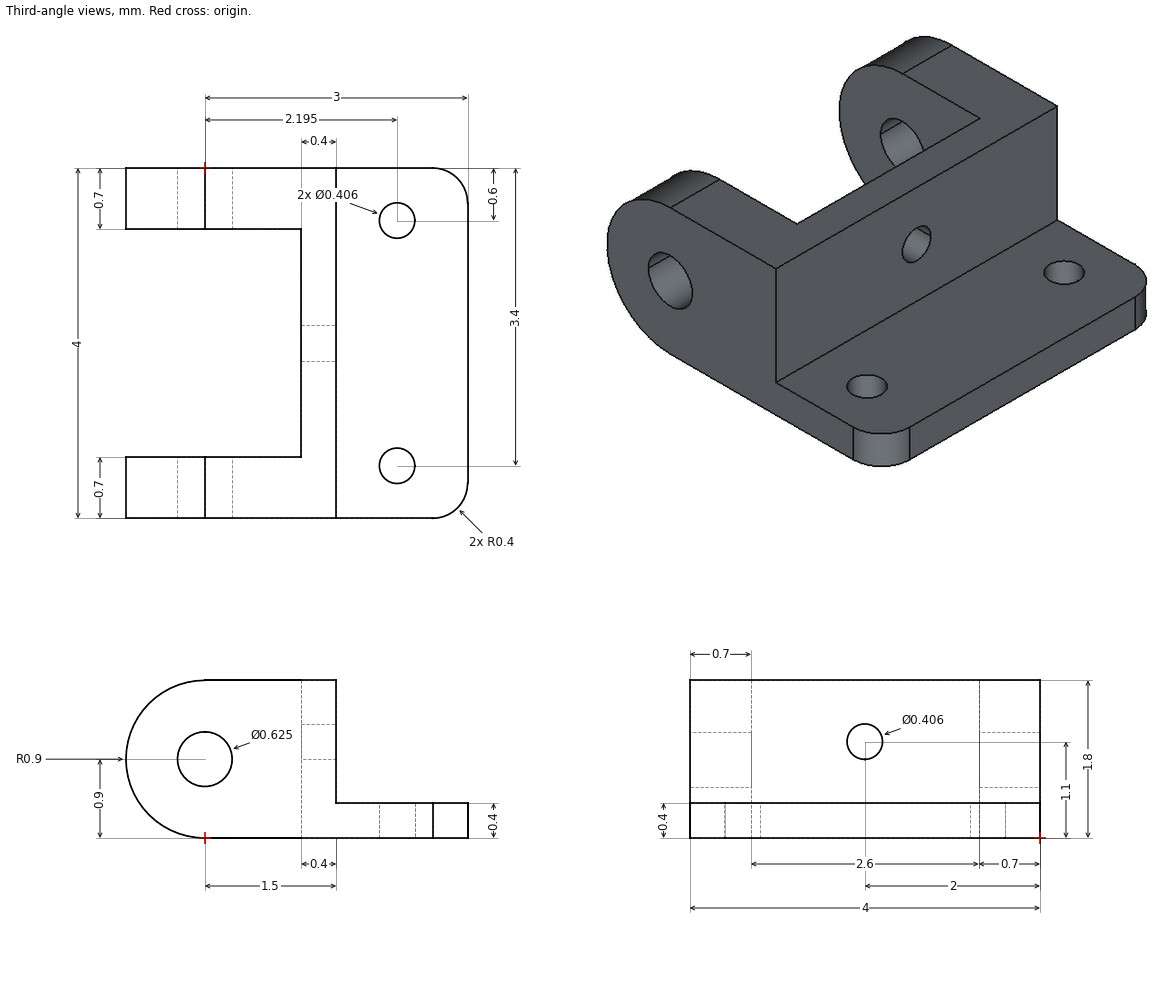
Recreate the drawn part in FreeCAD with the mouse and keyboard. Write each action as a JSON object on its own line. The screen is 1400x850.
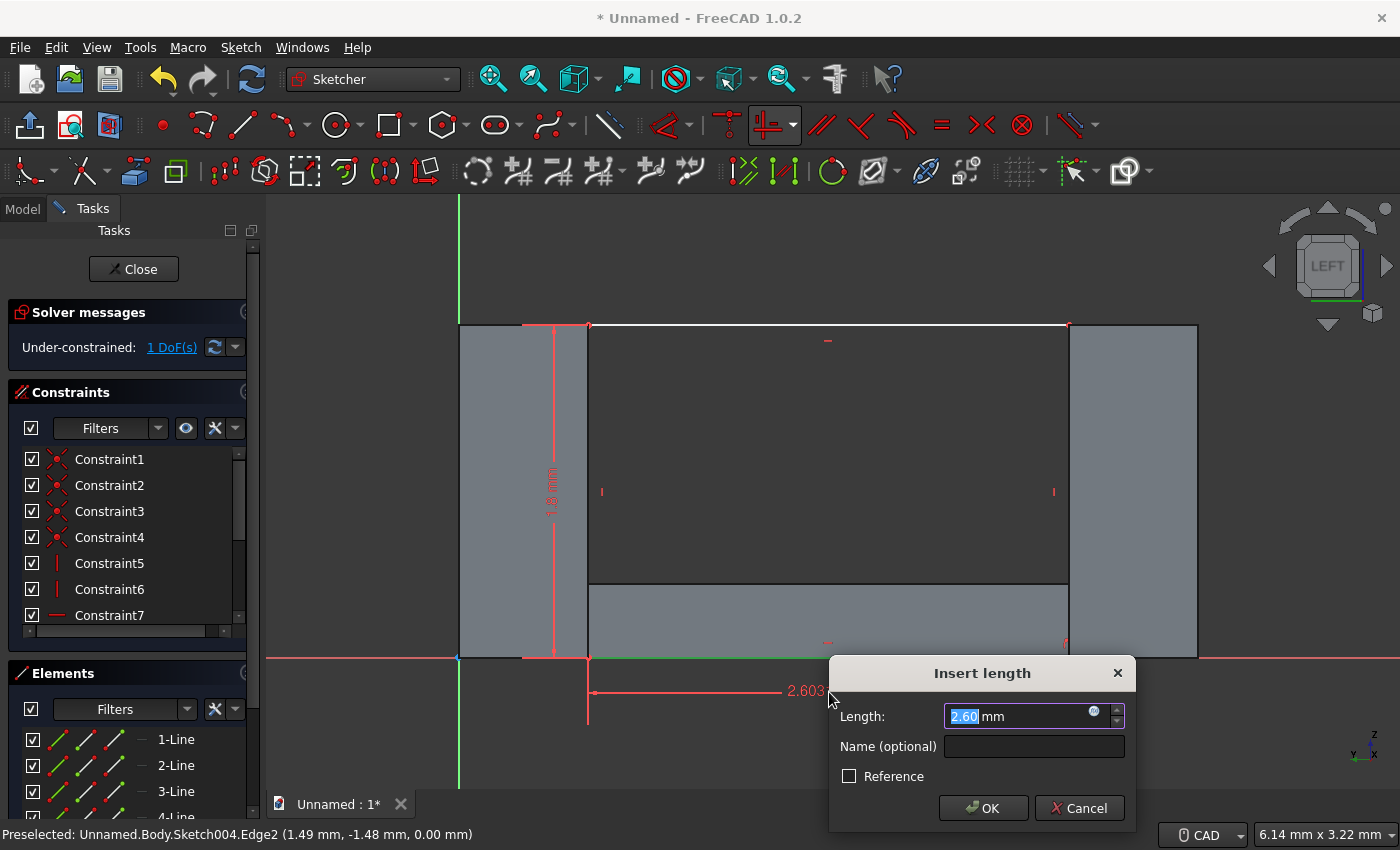
{"action": "type", "text": "2.6"}
{"action": "key", "text": "Return"}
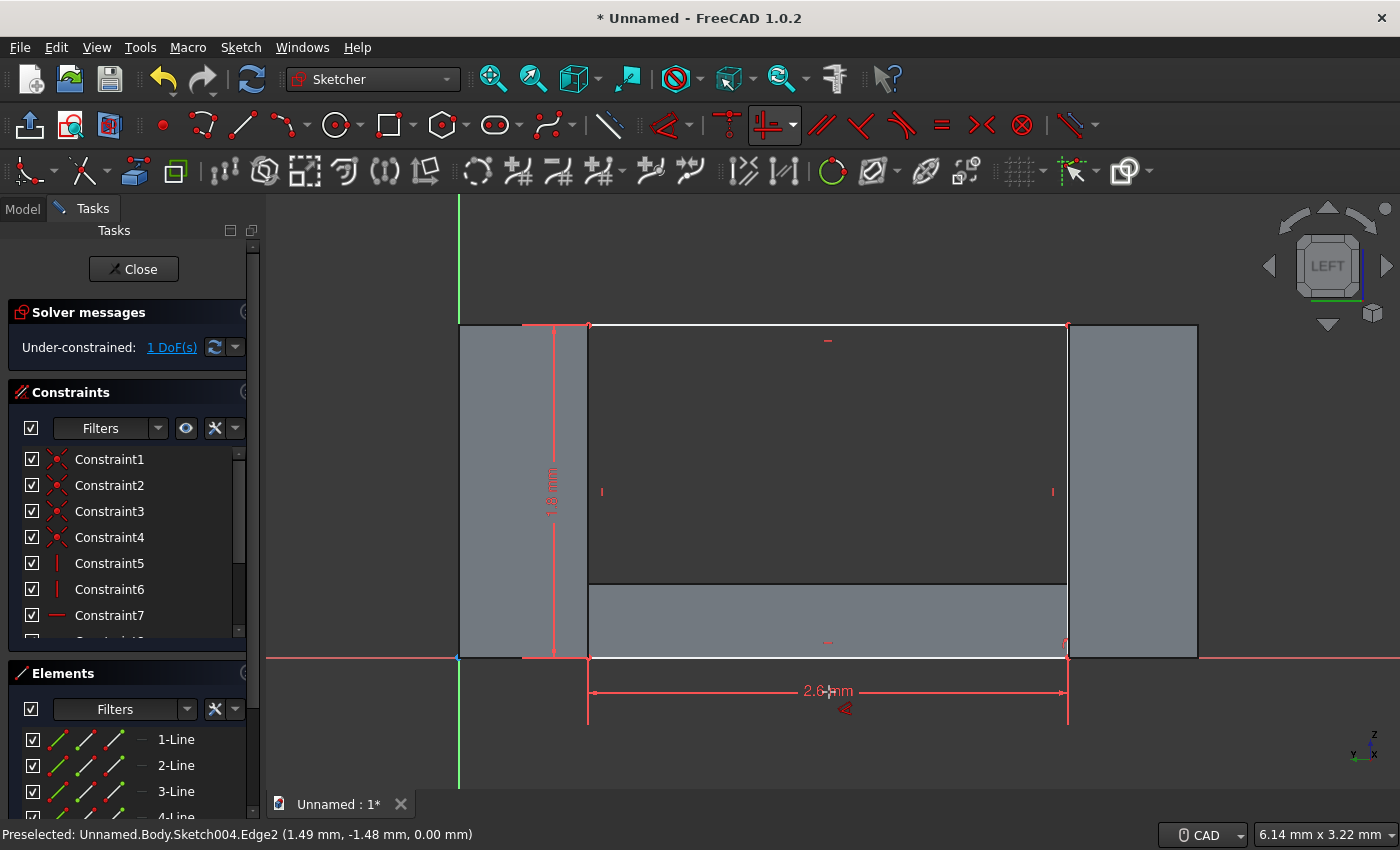
{"action": "left_click", "coordinate": [588, 325]}
{"action": "left_click", "coordinate": [523, 692]}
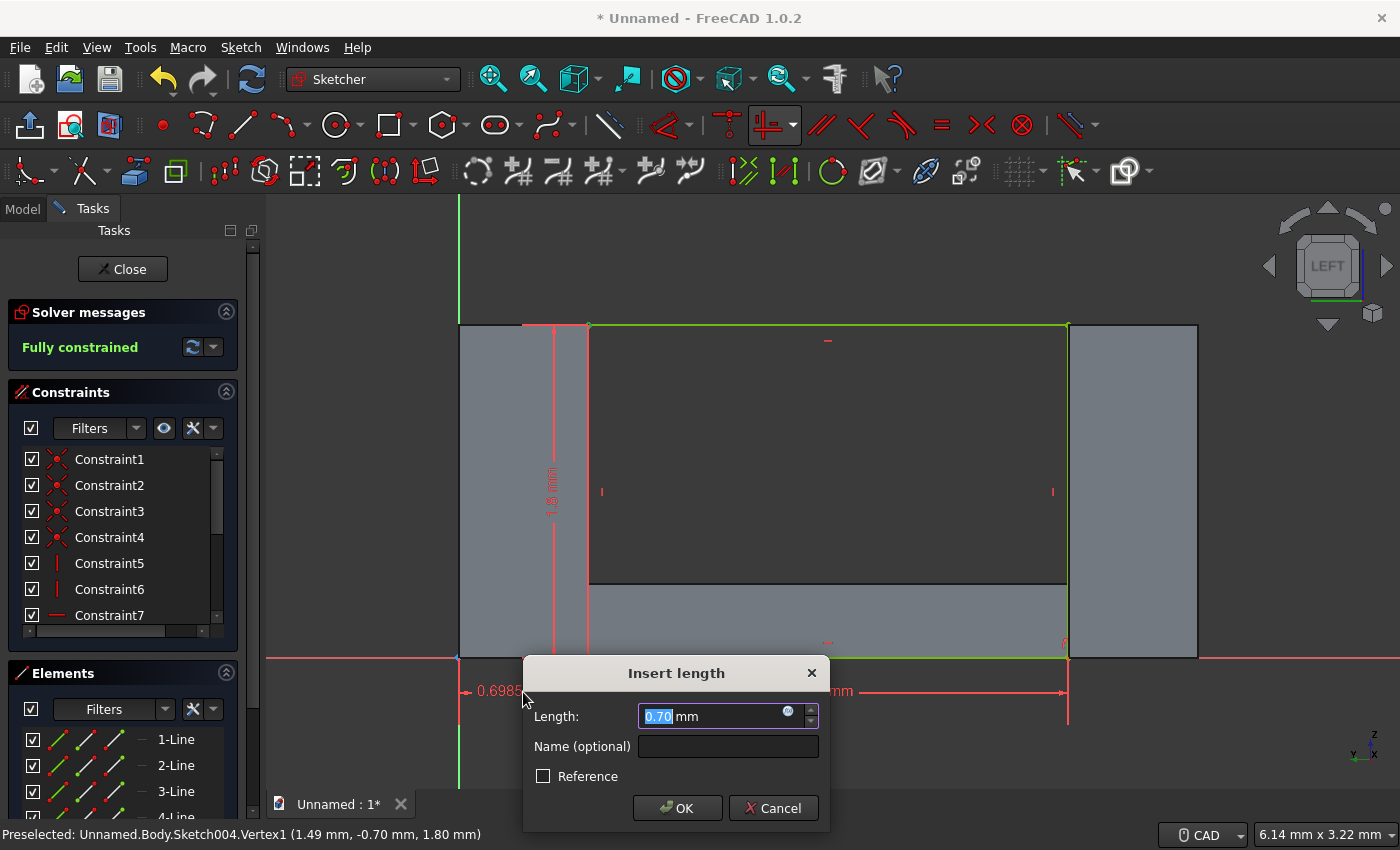
{"action": "type", "text": "0.7"}
{"action": "key", "text": "Return"}
{"action": "key", "text": "Escape"}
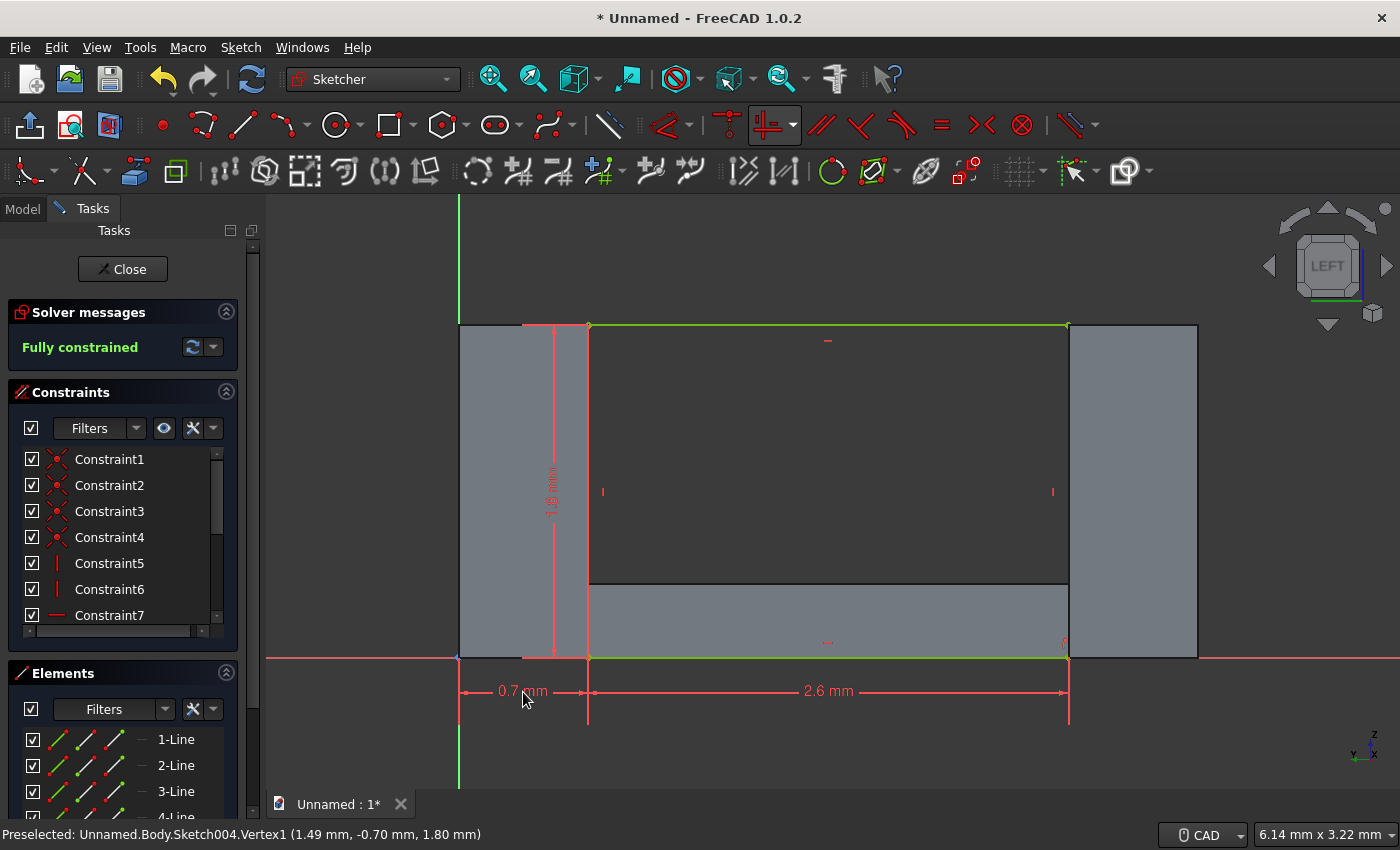
{"action": "left_click", "coordinate": [123, 269]}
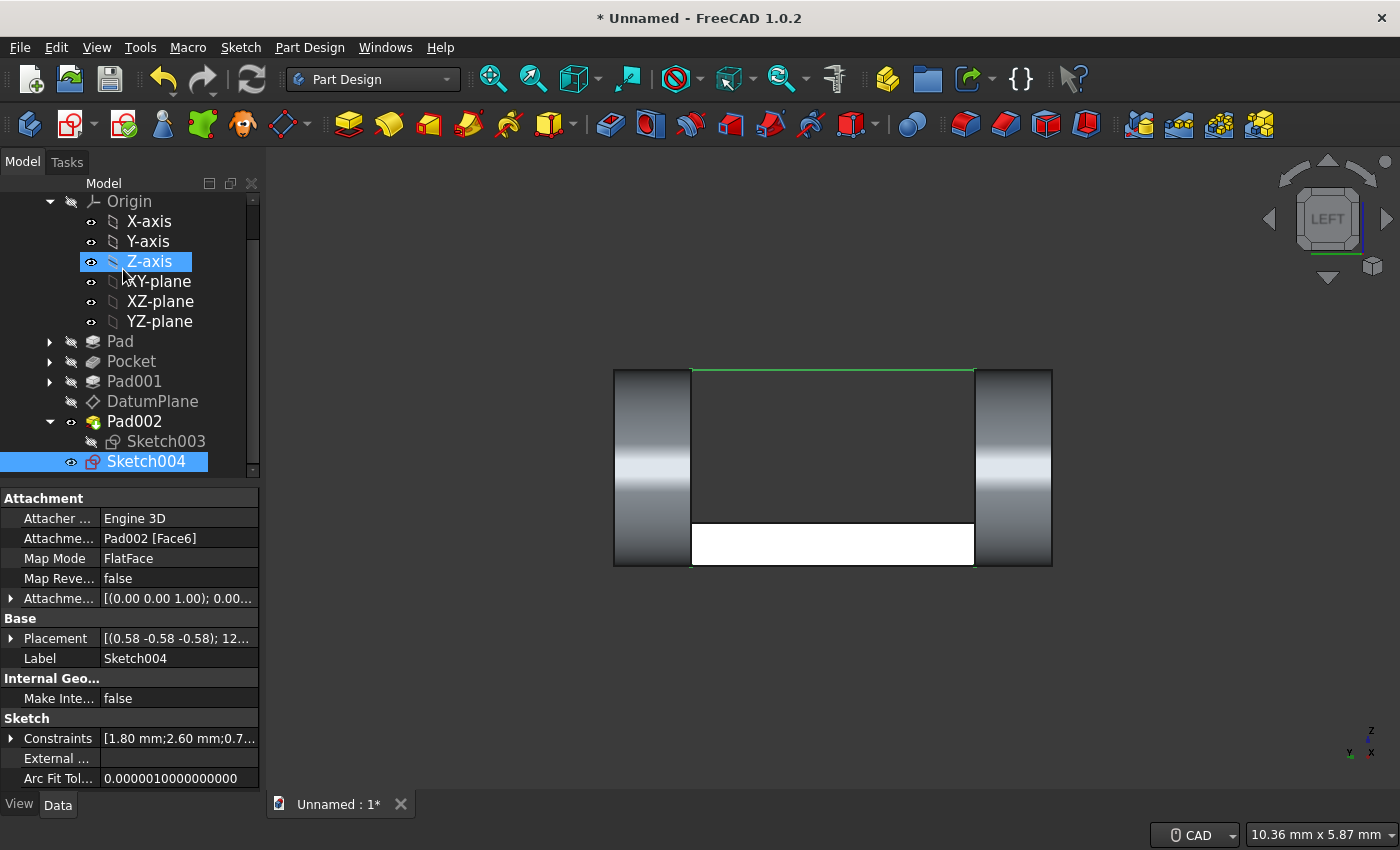
{"action": "left_click", "coordinate": [350, 124]}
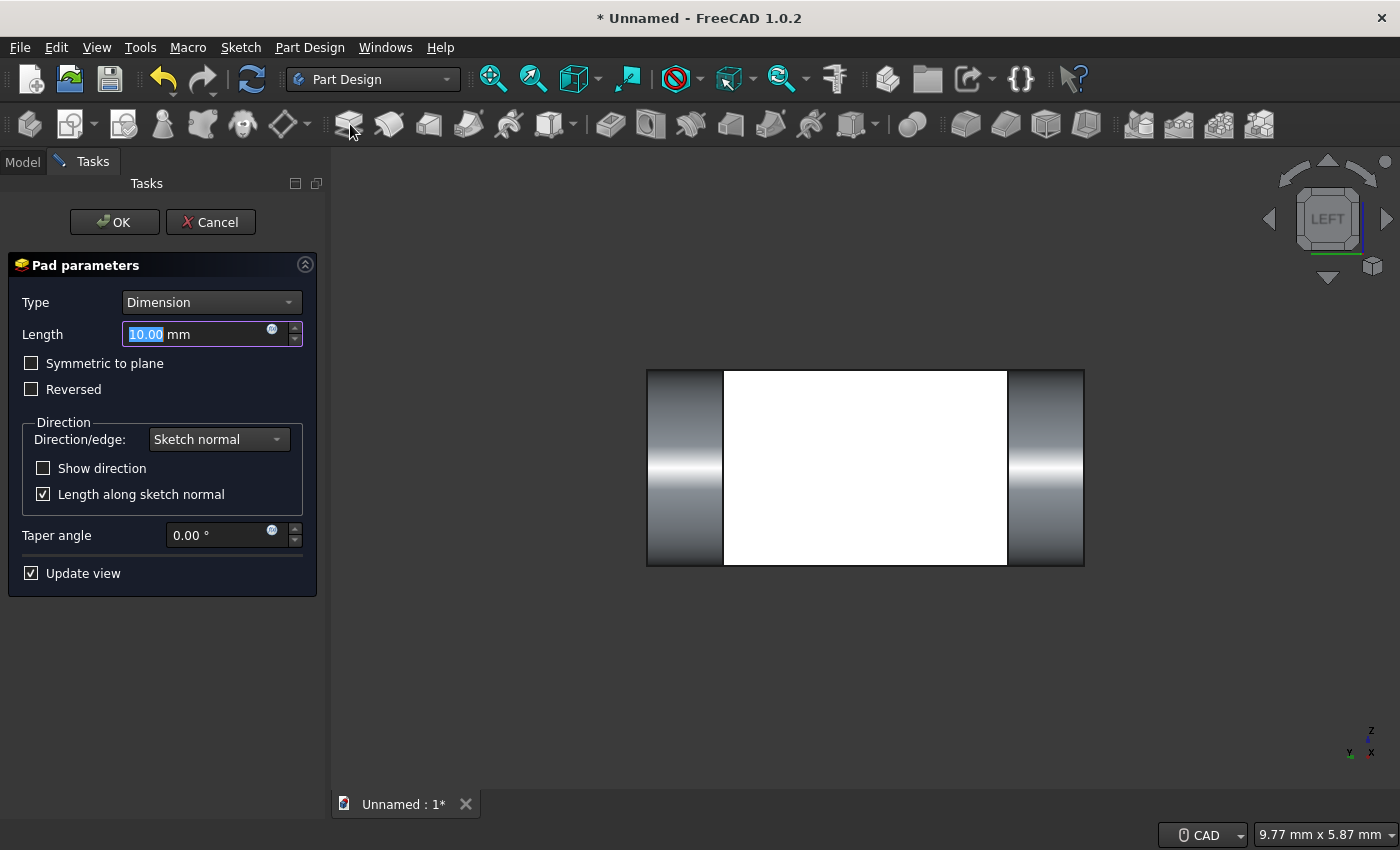
{"action": "type", "text": "0.4"}
{"action": "key", "text": "Tab"}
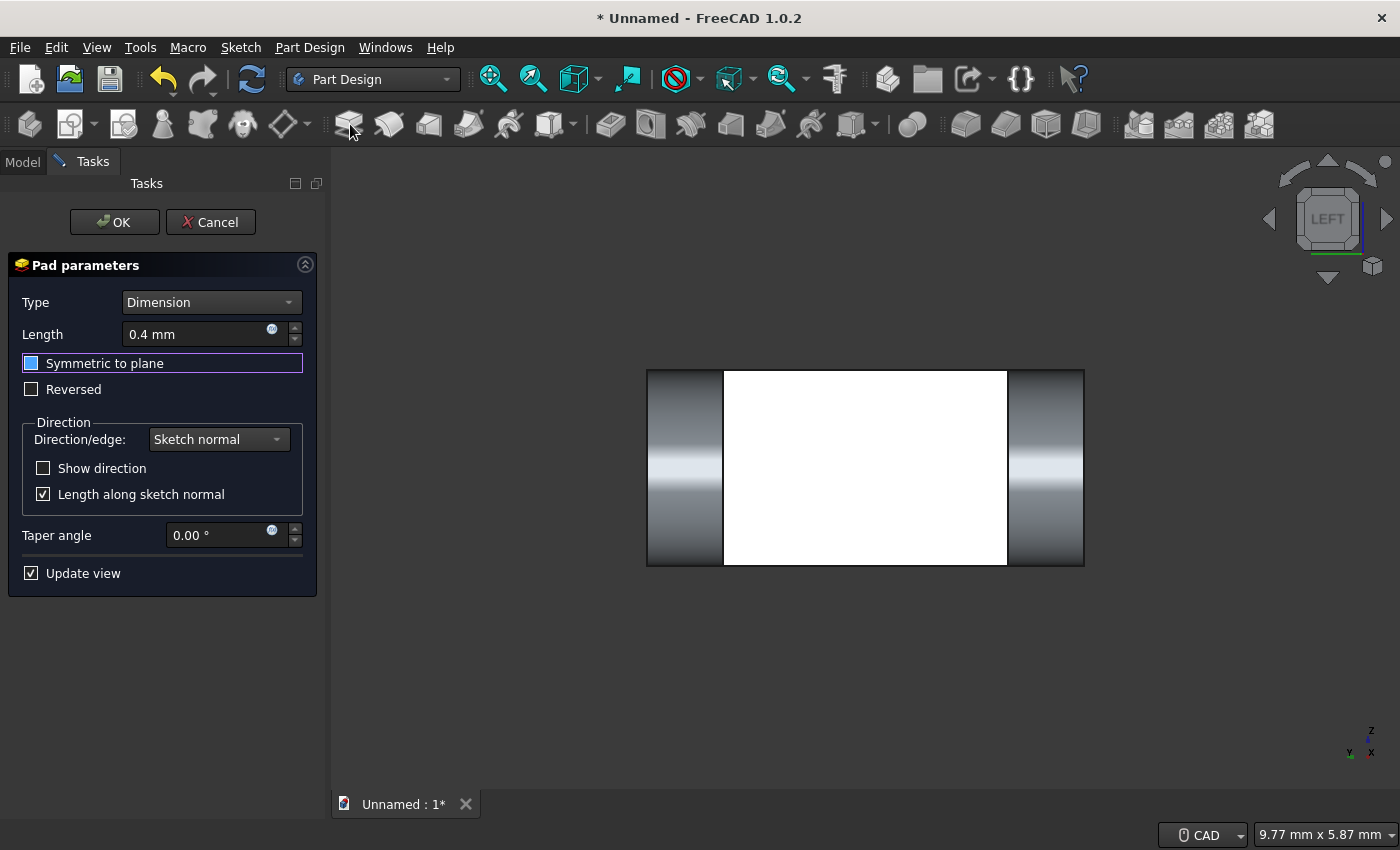
{"action": "left_click", "coordinate": [115, 222]}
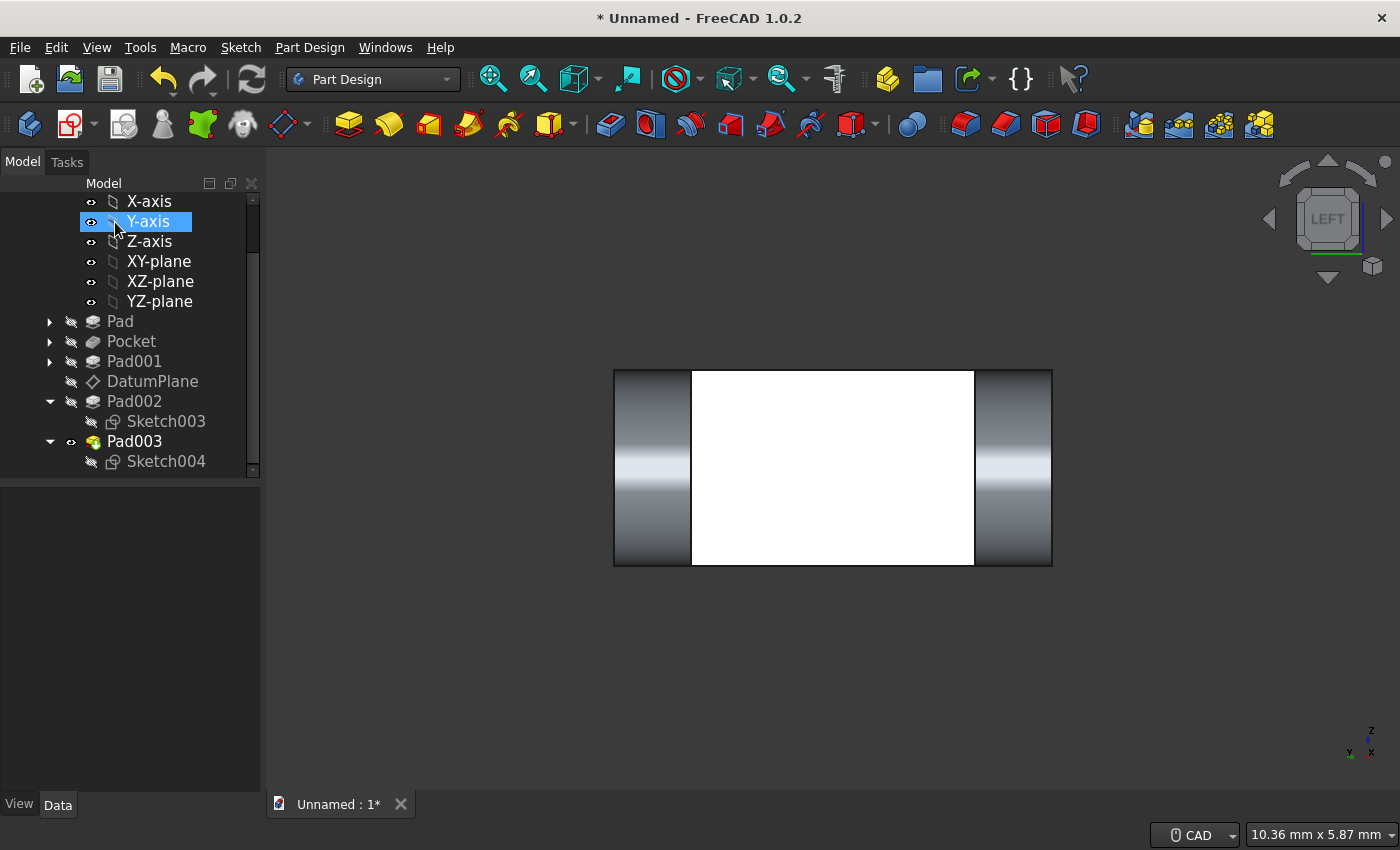
{"action": "key", "text": "v f"}